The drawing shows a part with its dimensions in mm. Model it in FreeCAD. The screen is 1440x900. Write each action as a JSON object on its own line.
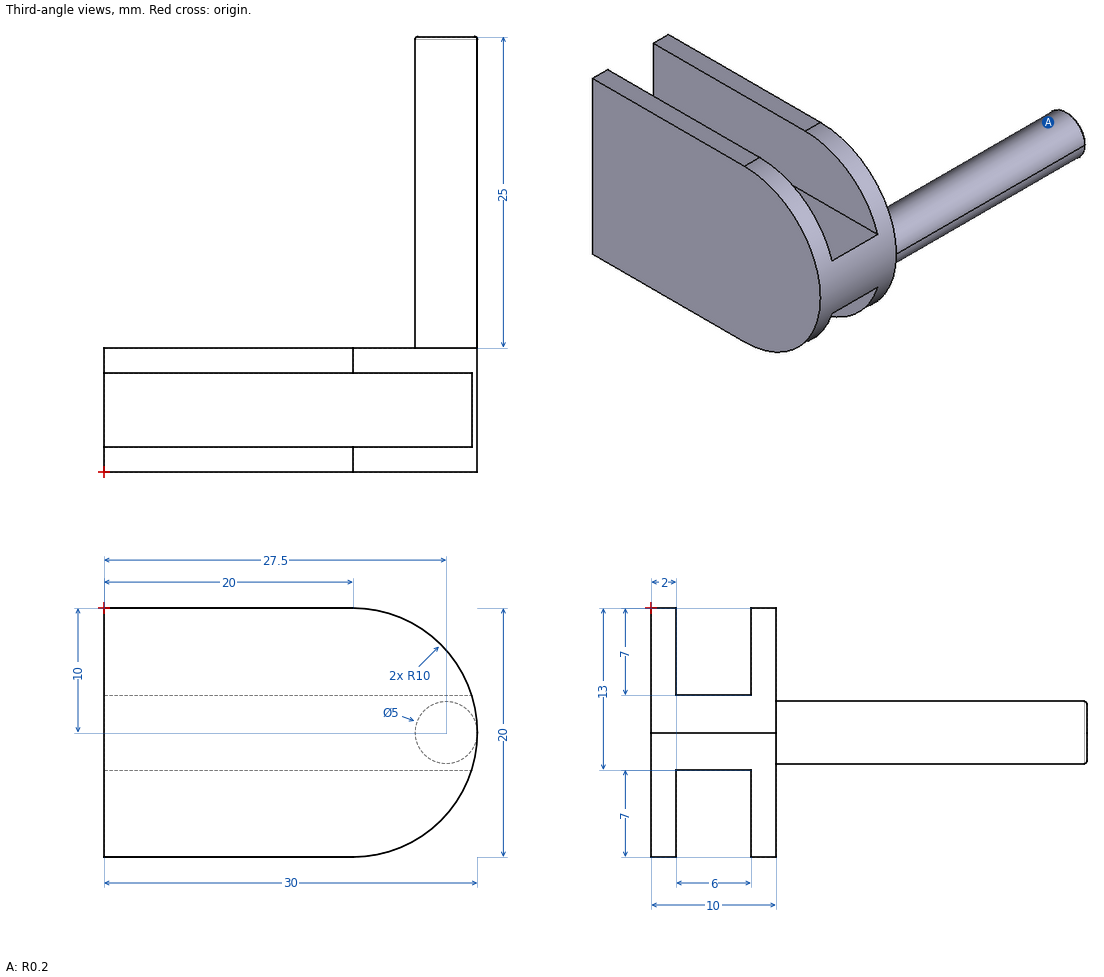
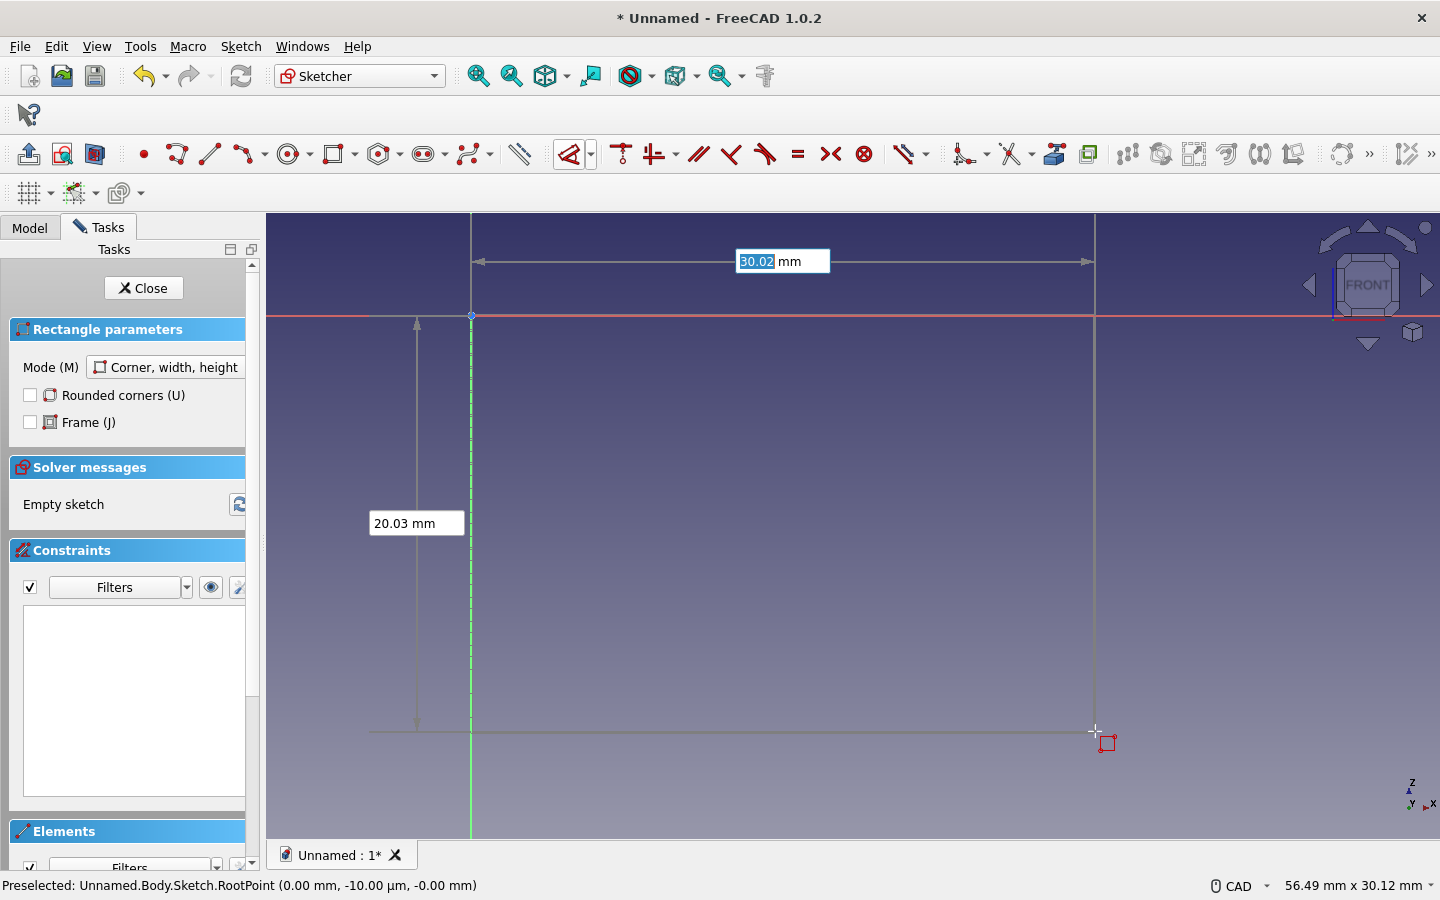
{"action": "type", "text": "30"}
{"action": "key", "text": "Tab"}
{"action": "type", "text": "20"}
{"action": "key", "text": "Return"}
{"action": "key", "text": "Escape"}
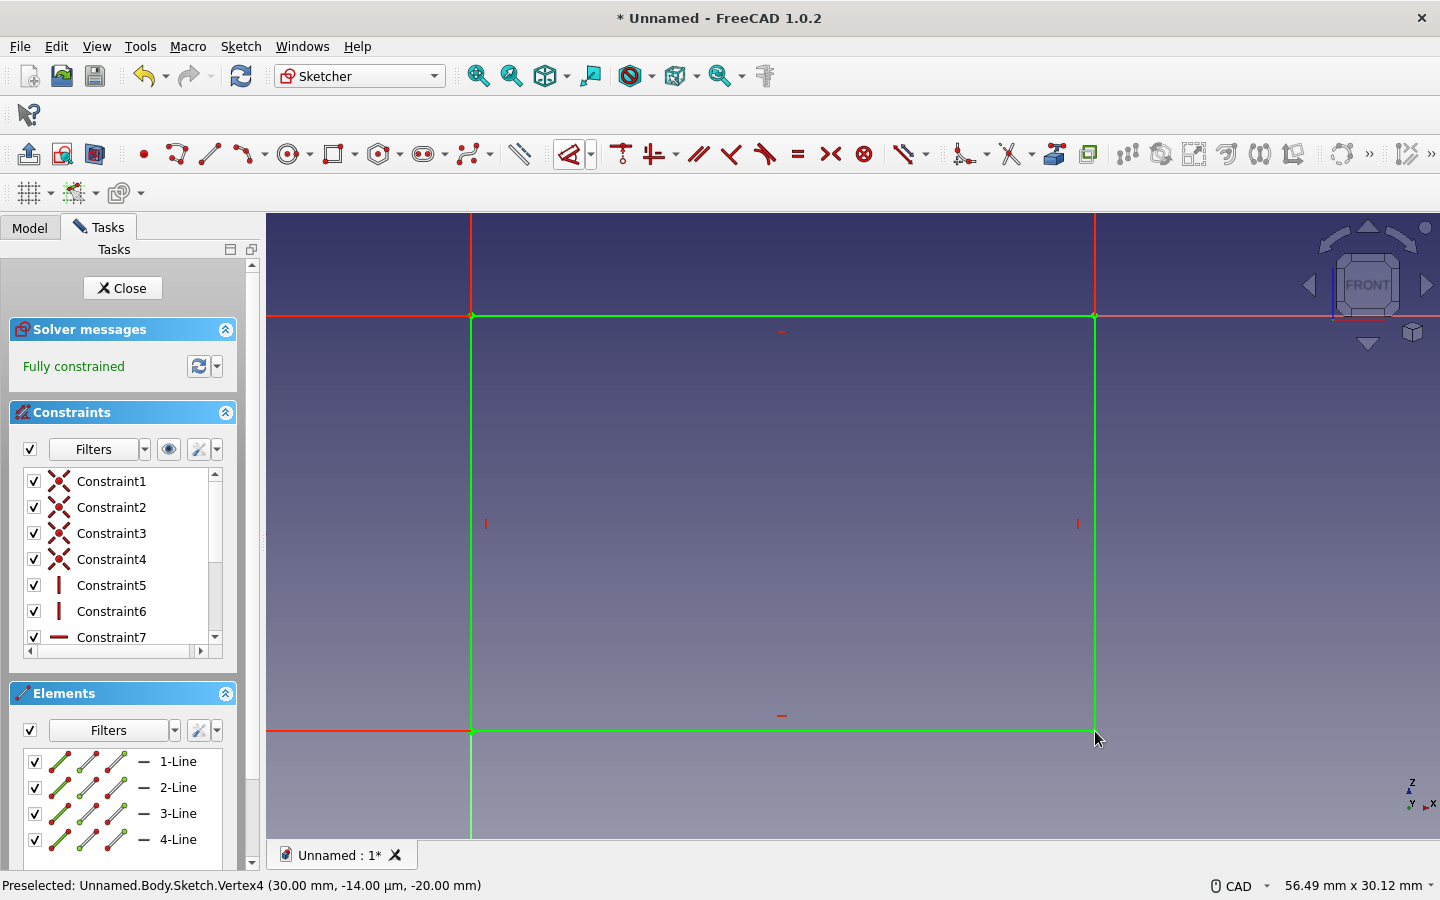
{"action": "left_click", "coordinate": [123, 288]}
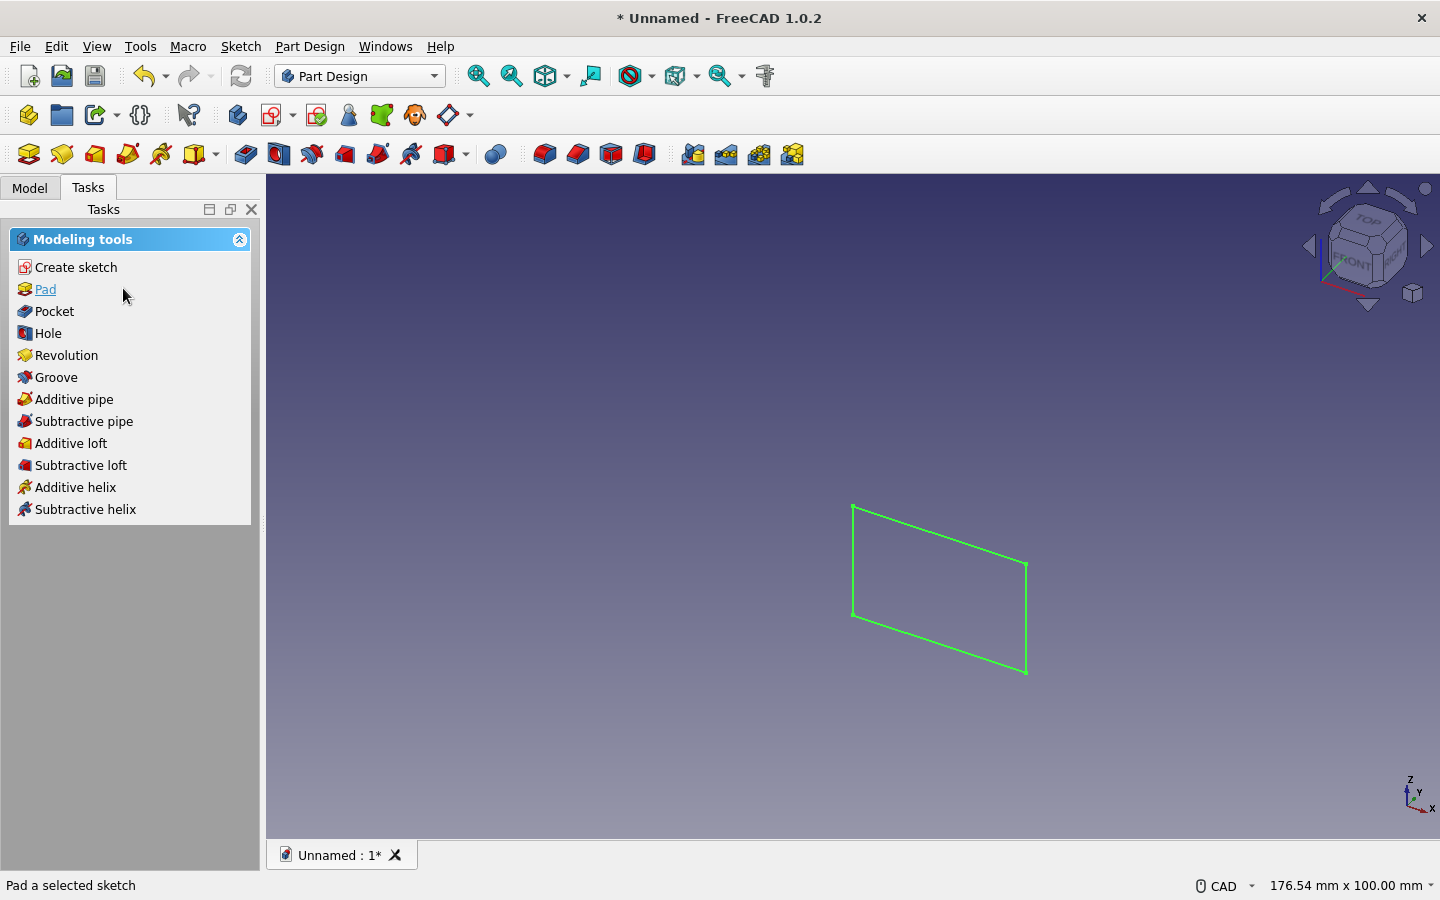
{"action": "left_click", "coordinate": [29, 154]}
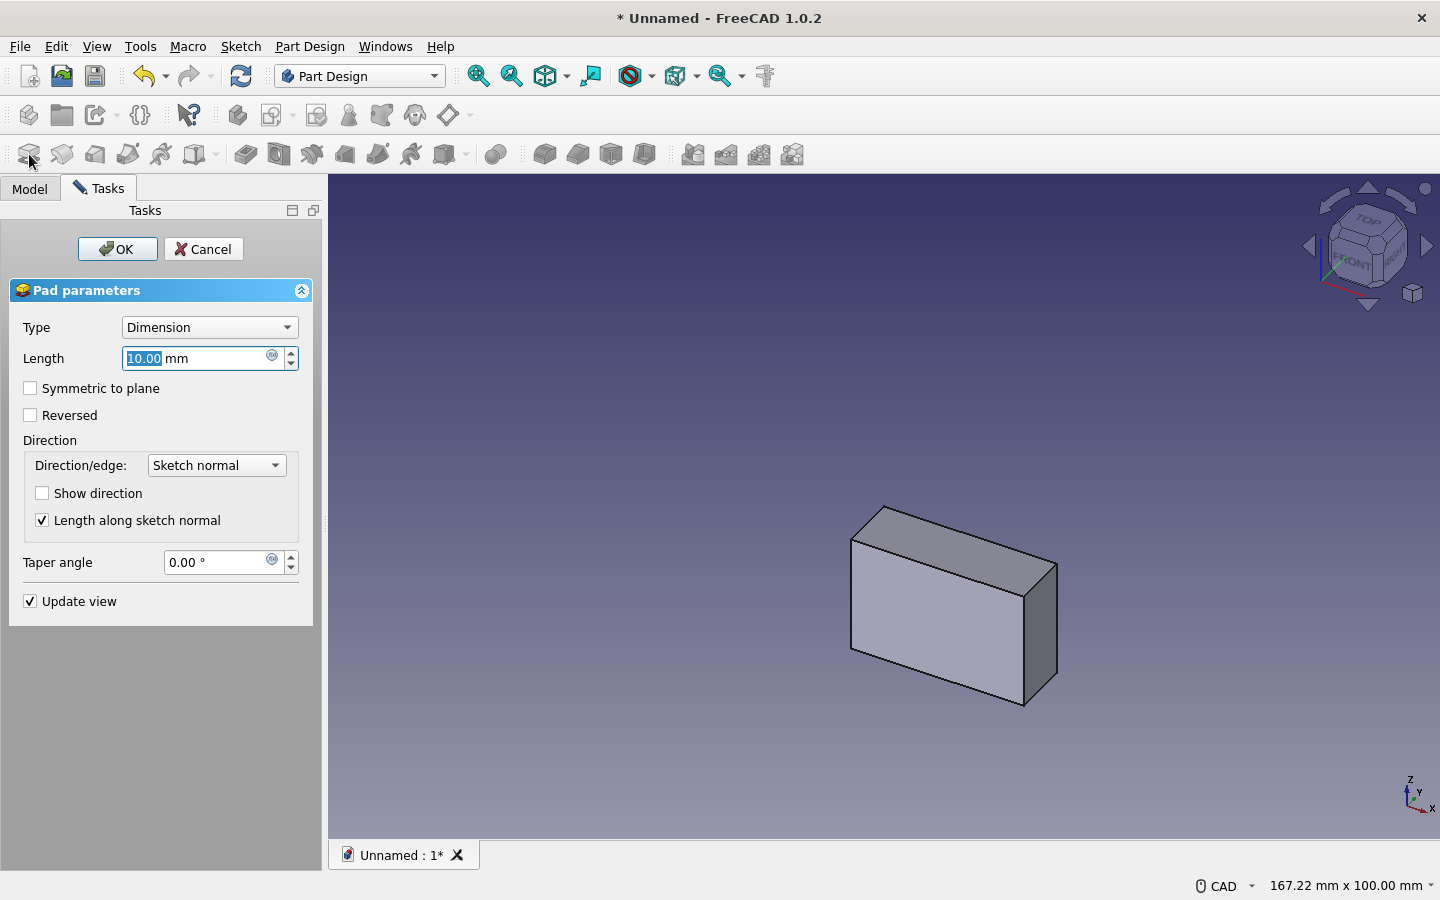
{"action": "type", "text": "10"}
{"action": "key", "text": "Tab"}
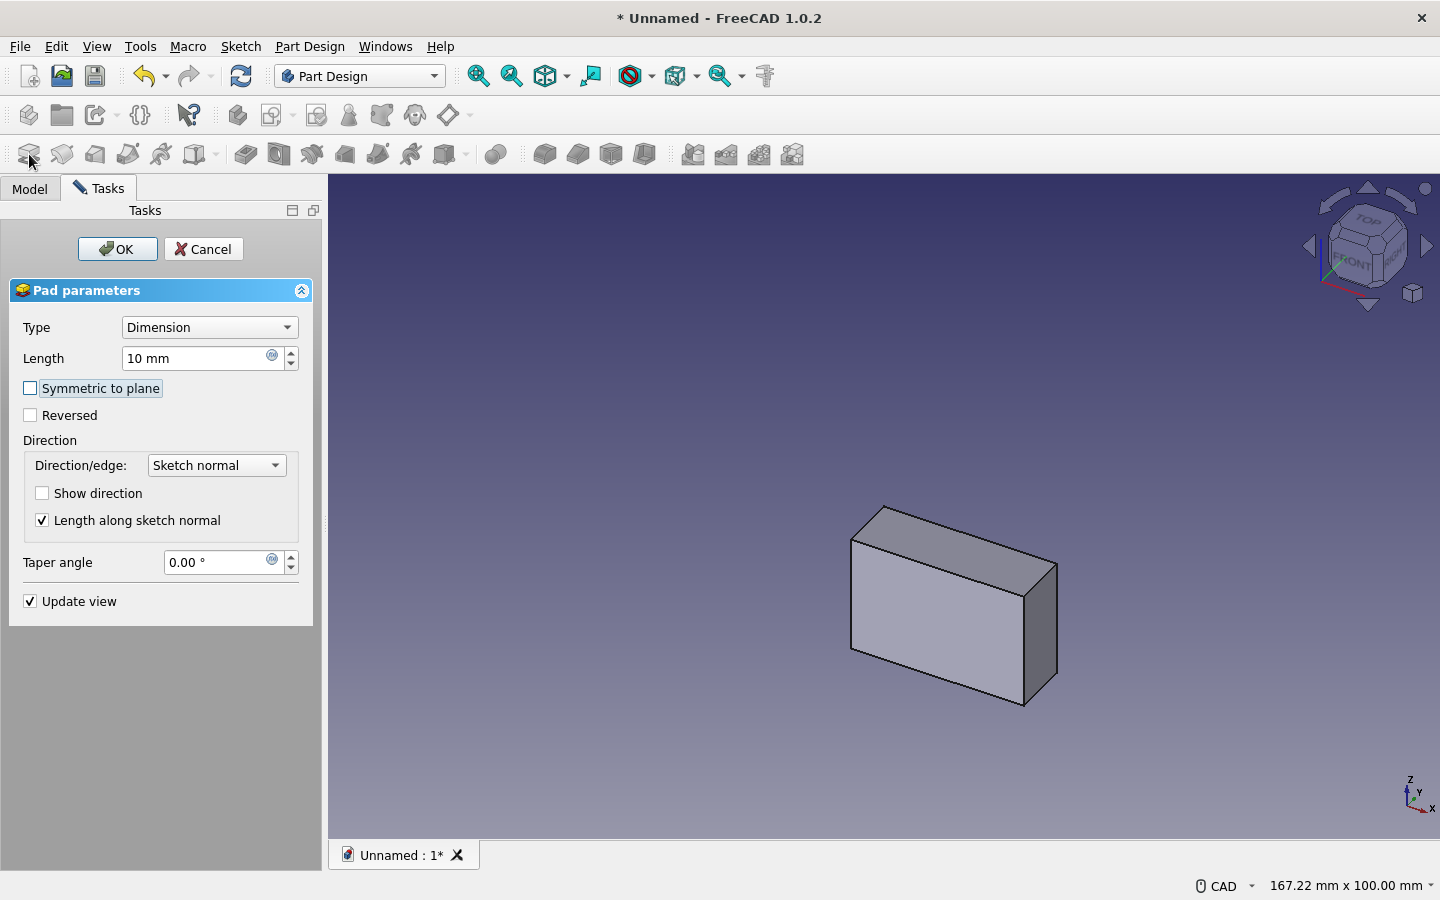
{"action": "left_click", "coordinate": [31, 415]}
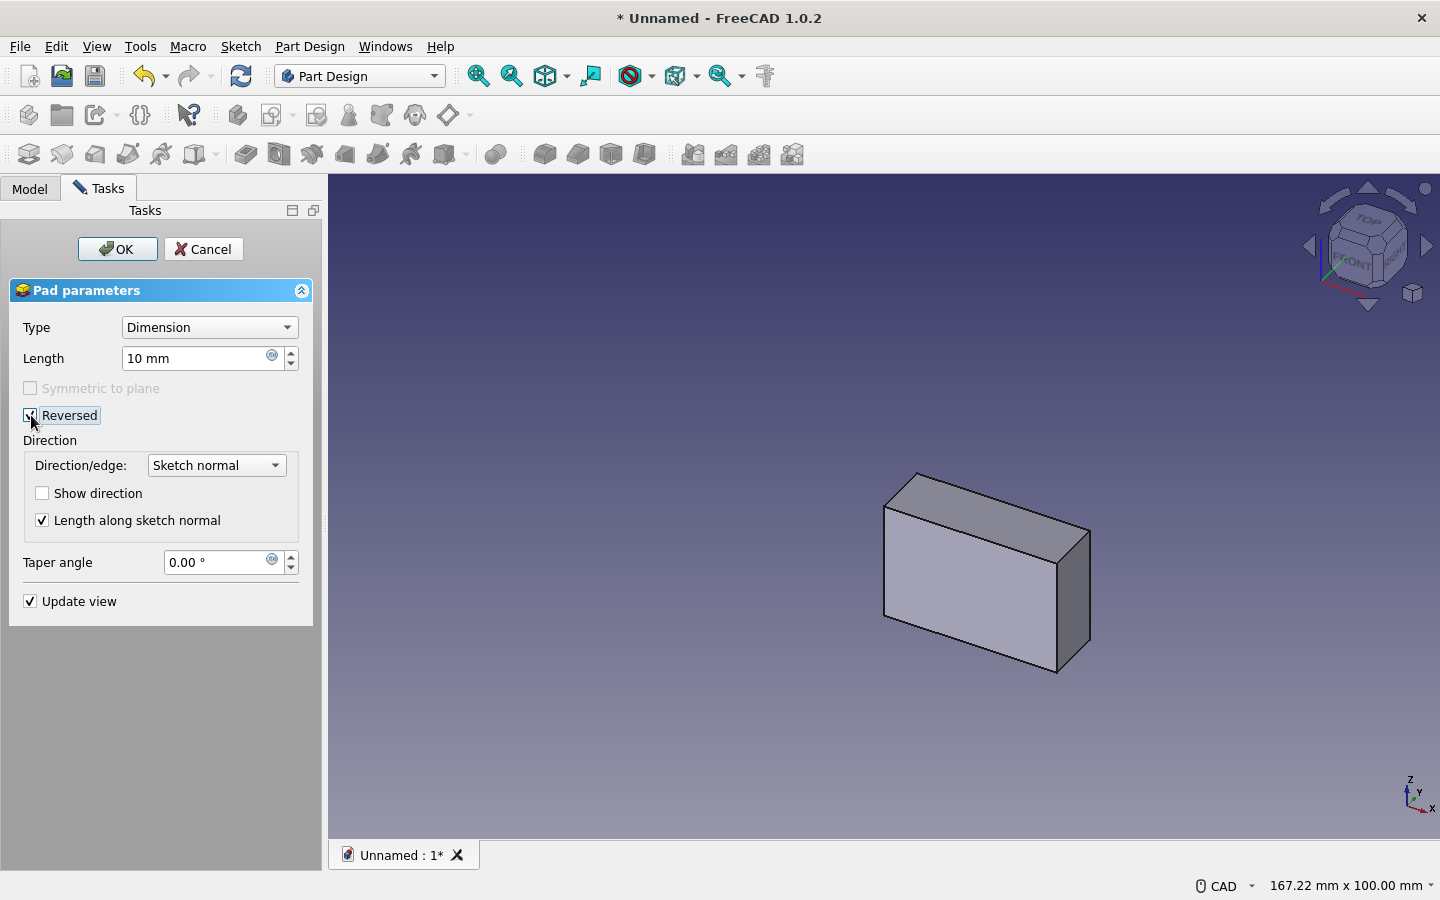
{"action": "left_click", "coordinate": [118, 249]}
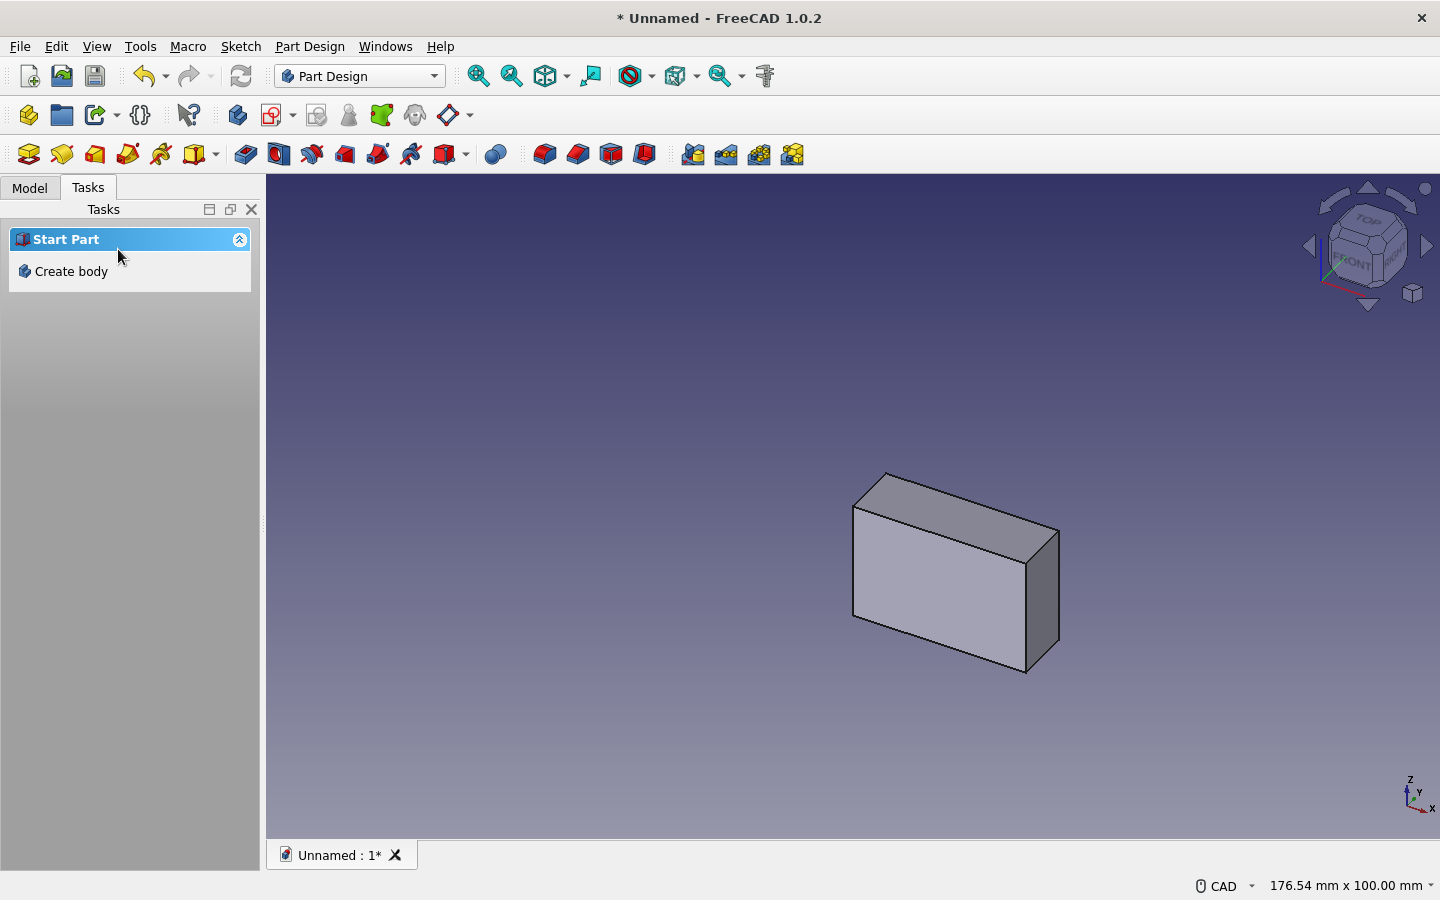
{"action": "left_click", "coordinate": [479, 76]}